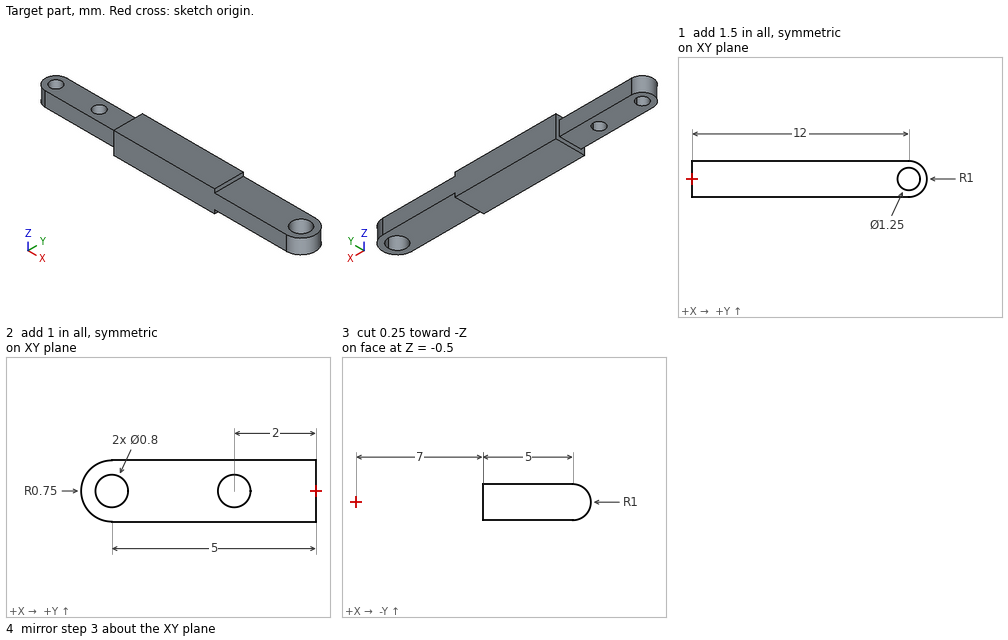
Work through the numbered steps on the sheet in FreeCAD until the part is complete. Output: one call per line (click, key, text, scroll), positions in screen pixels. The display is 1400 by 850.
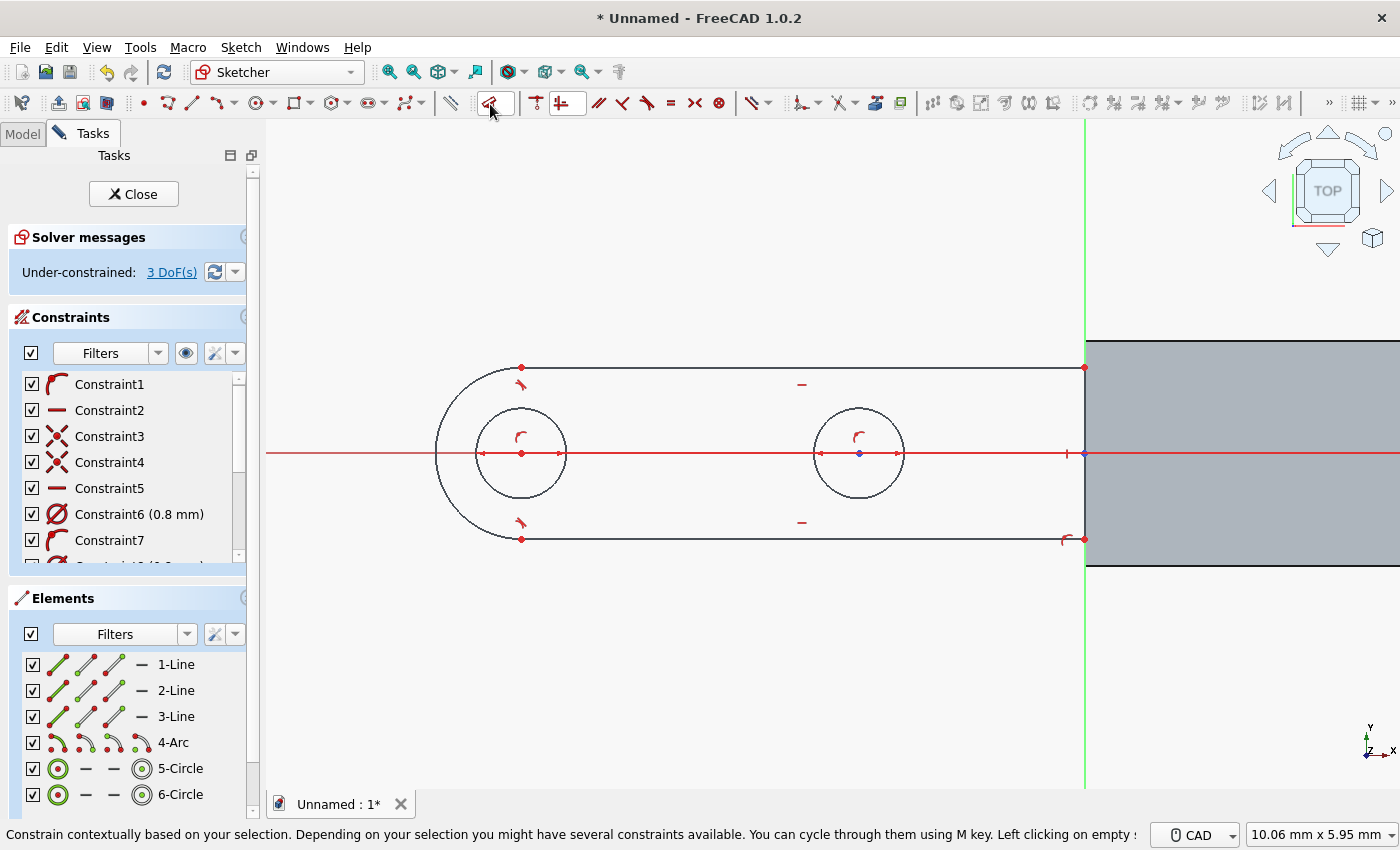
click(452, 403)
click(426, 384)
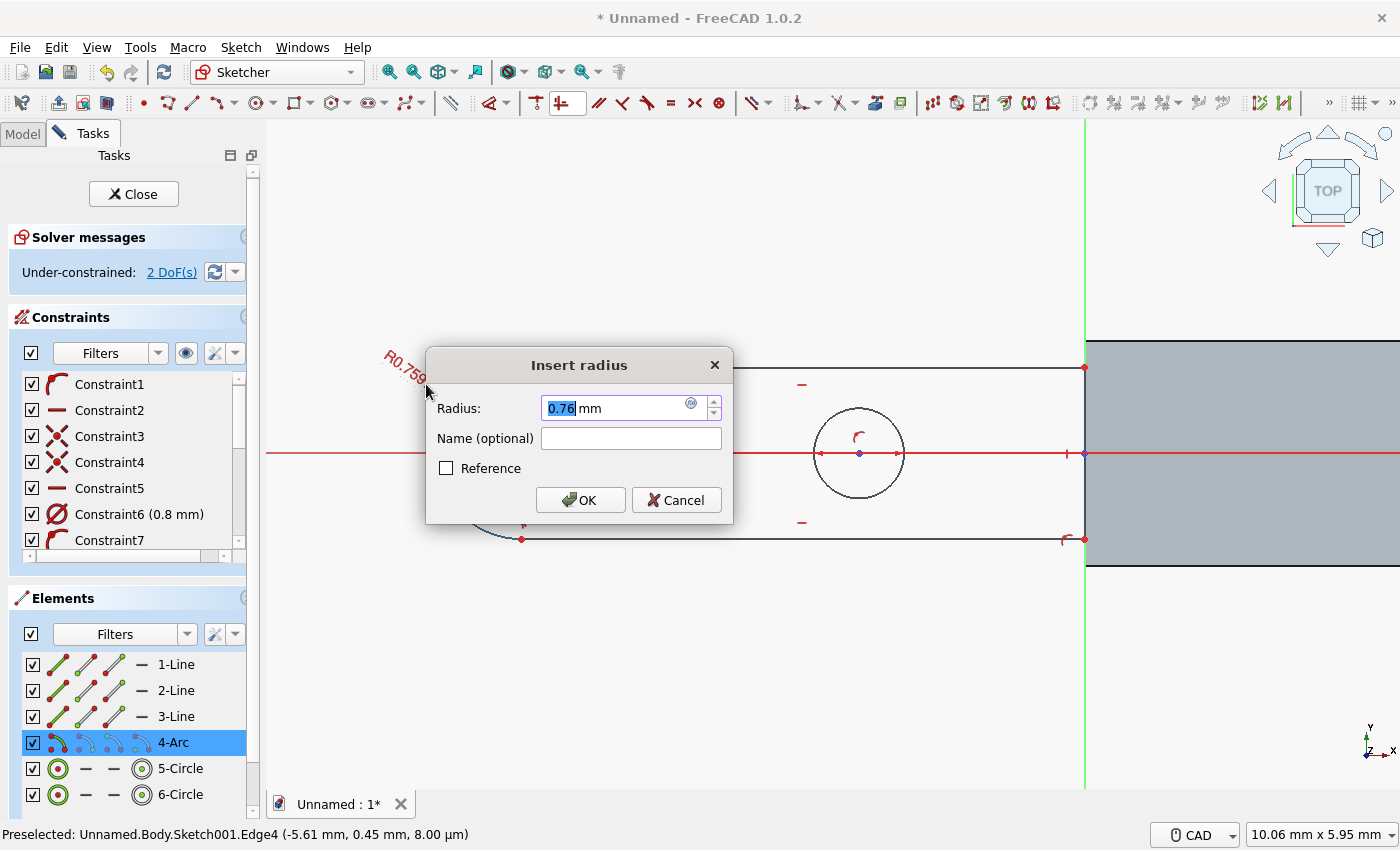
text(0.75)
key(Return)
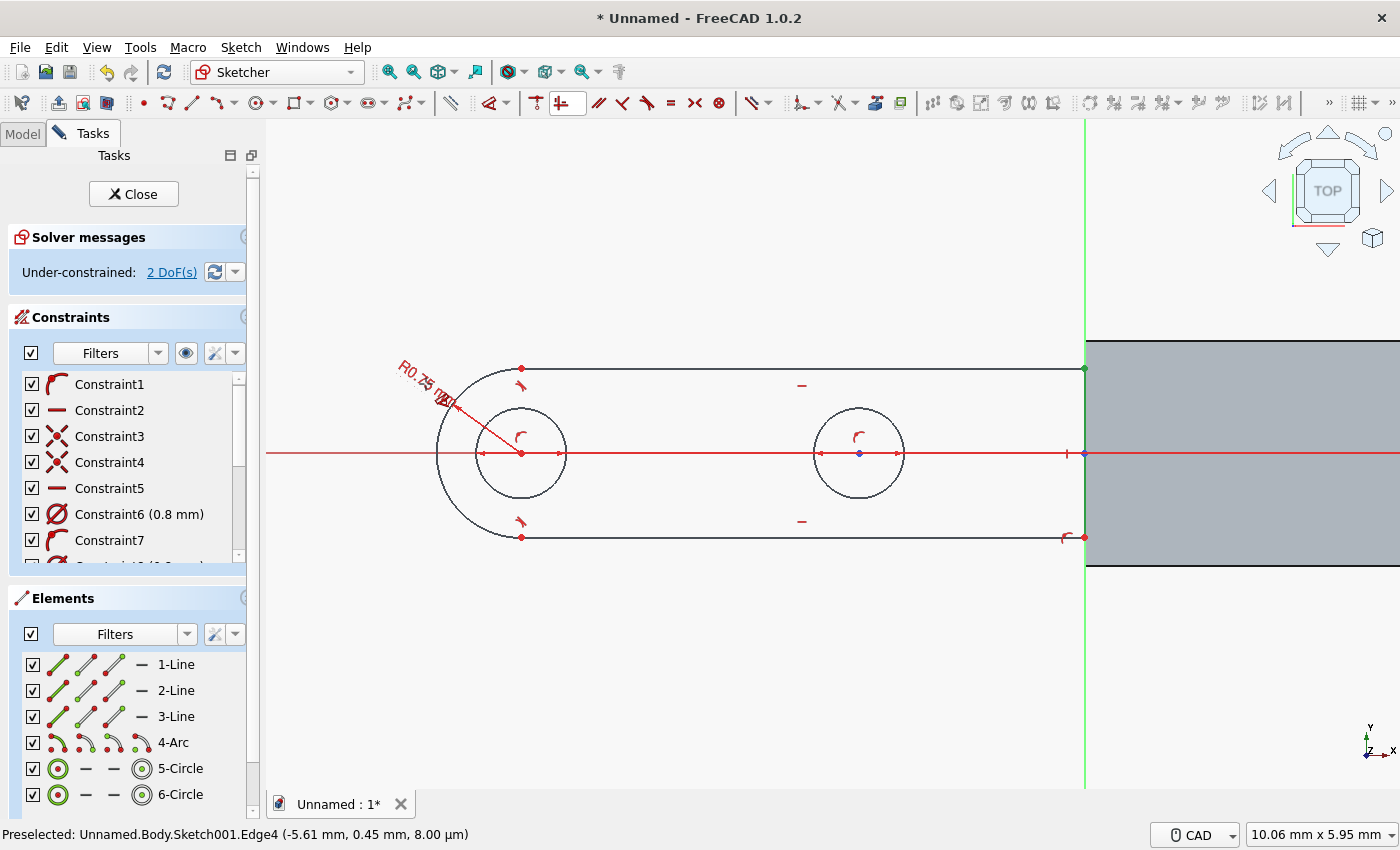
click(690, 538)
click(803, 572)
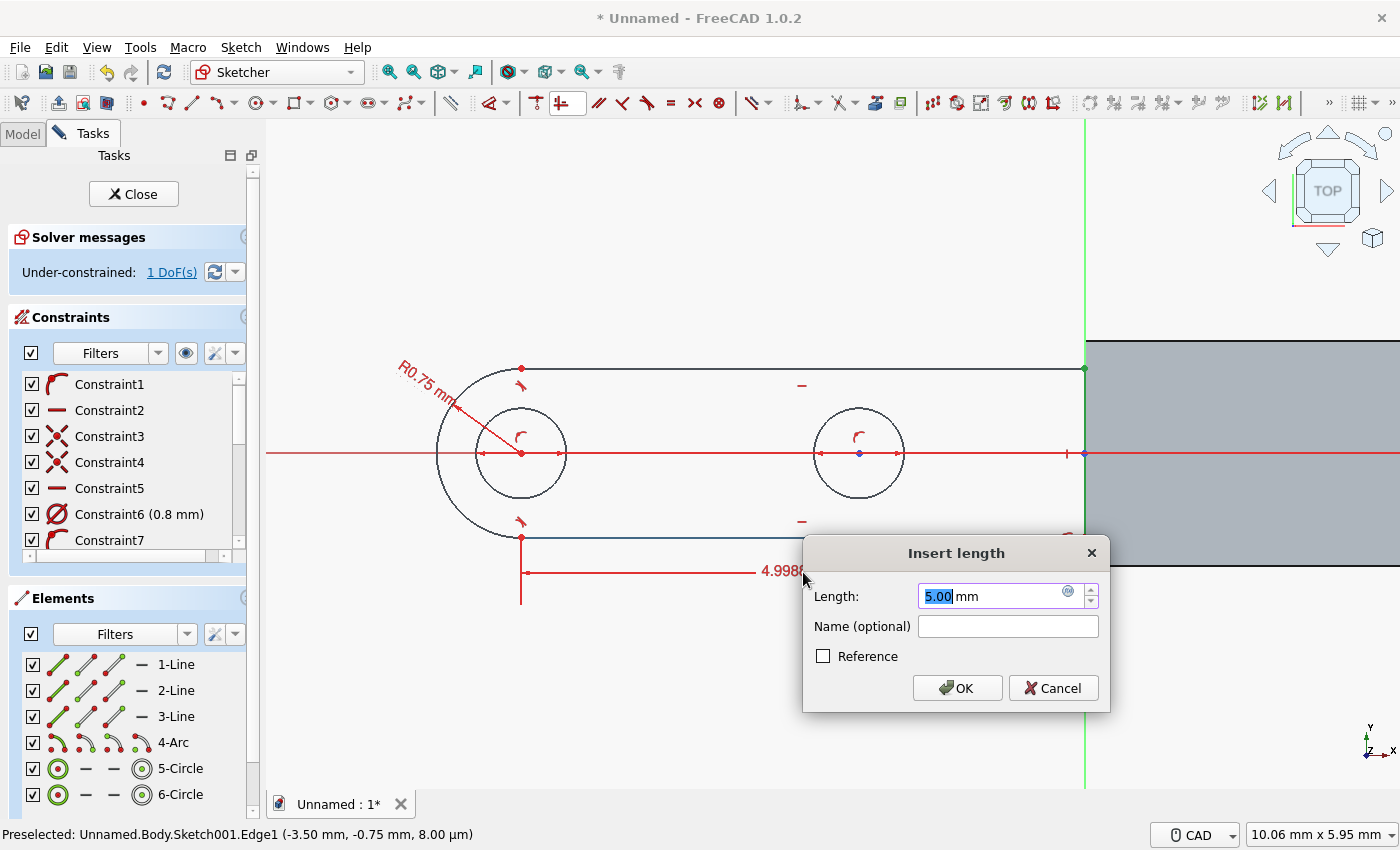
text(5)
key(Return)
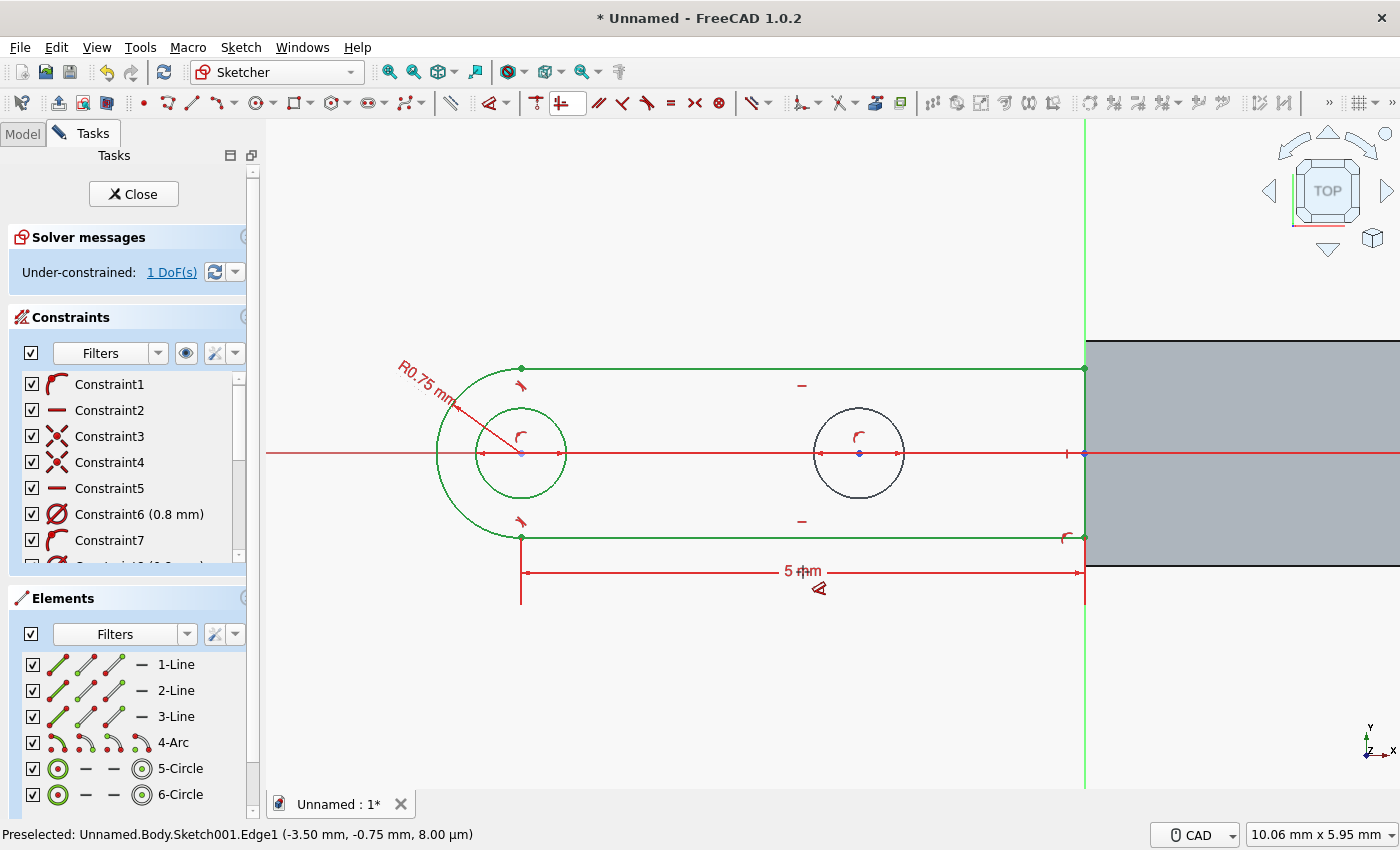
click(859, 453)
click(972, 487)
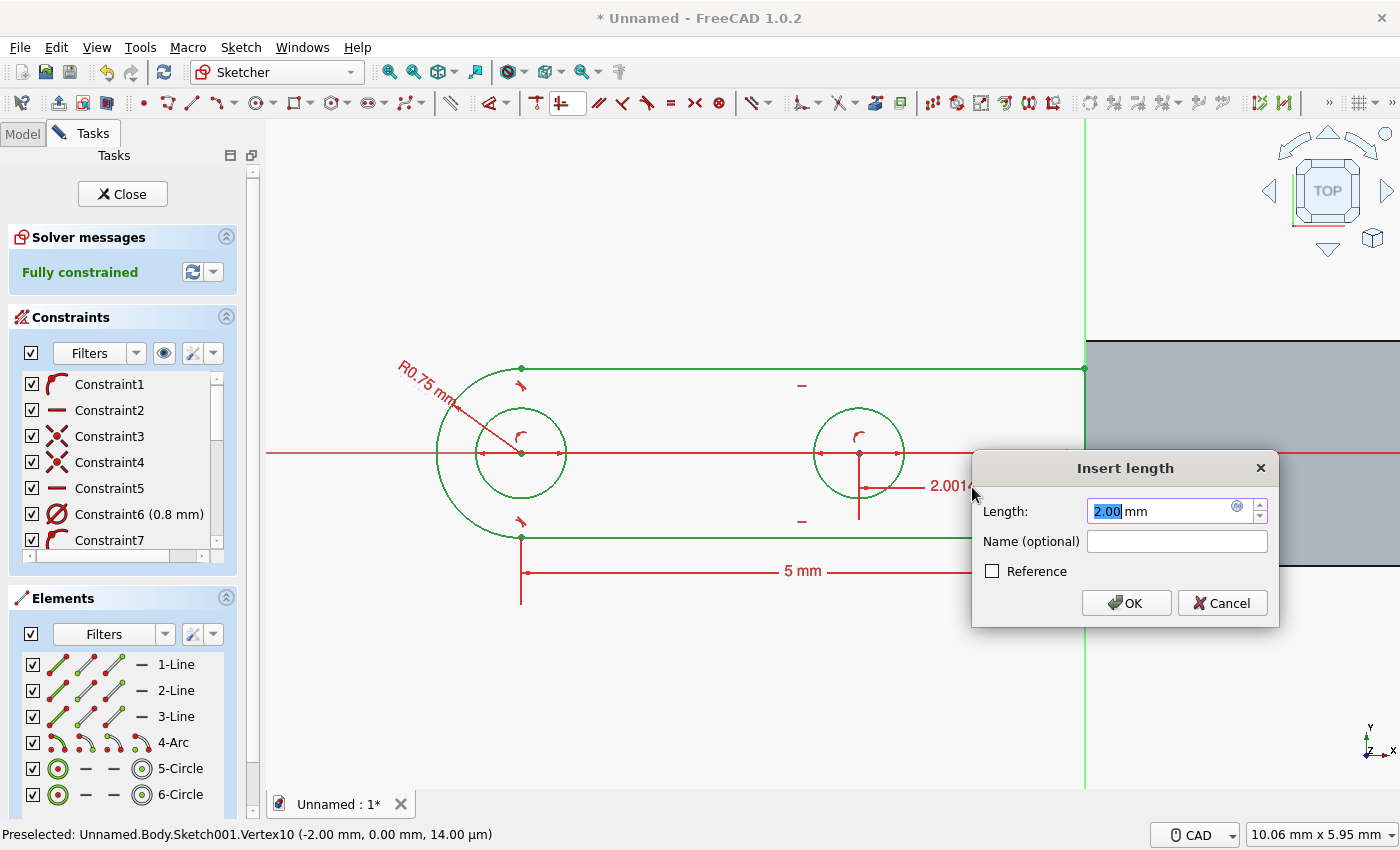
text(2)
key(Return)
key(Escape)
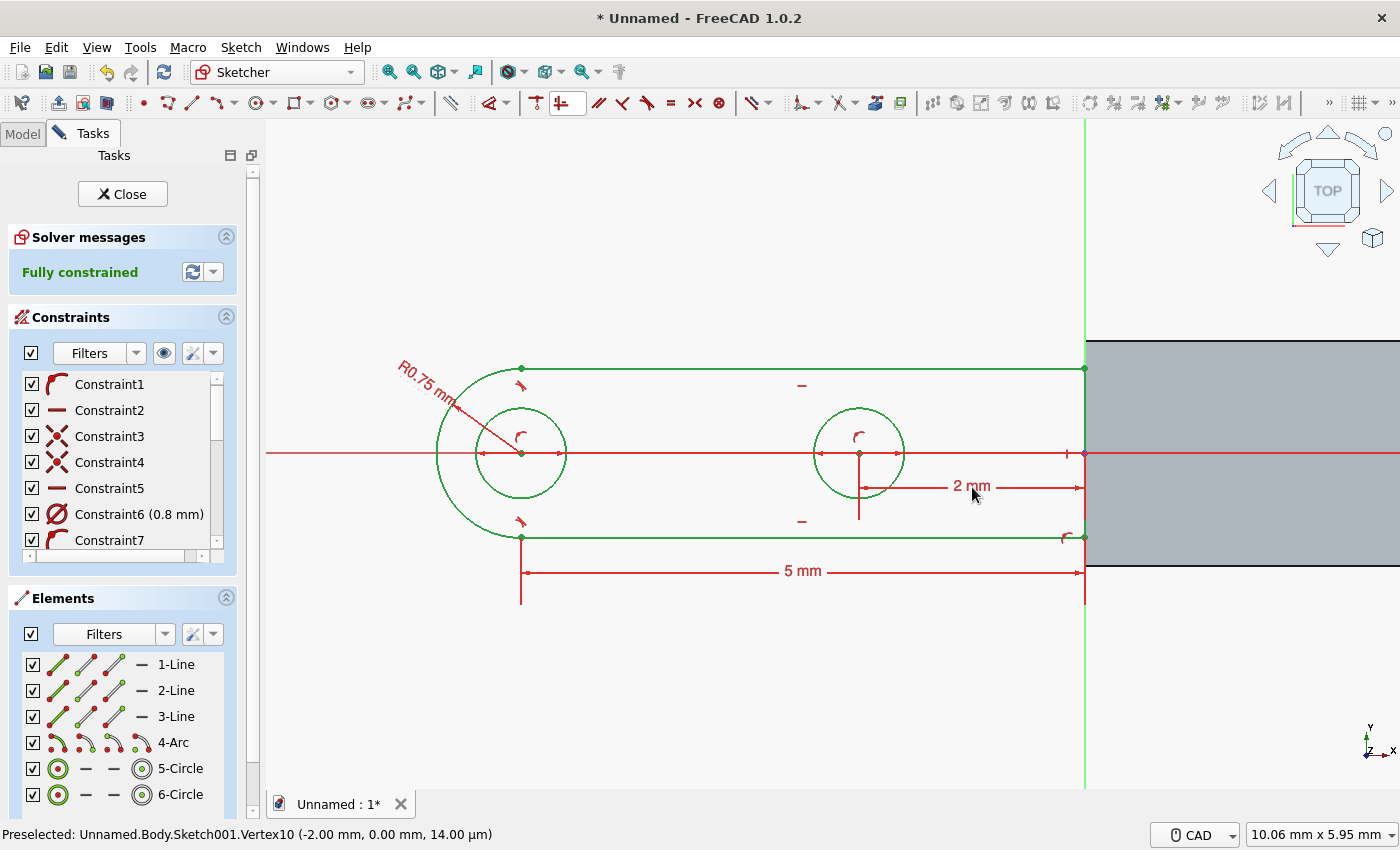
click(123, 194)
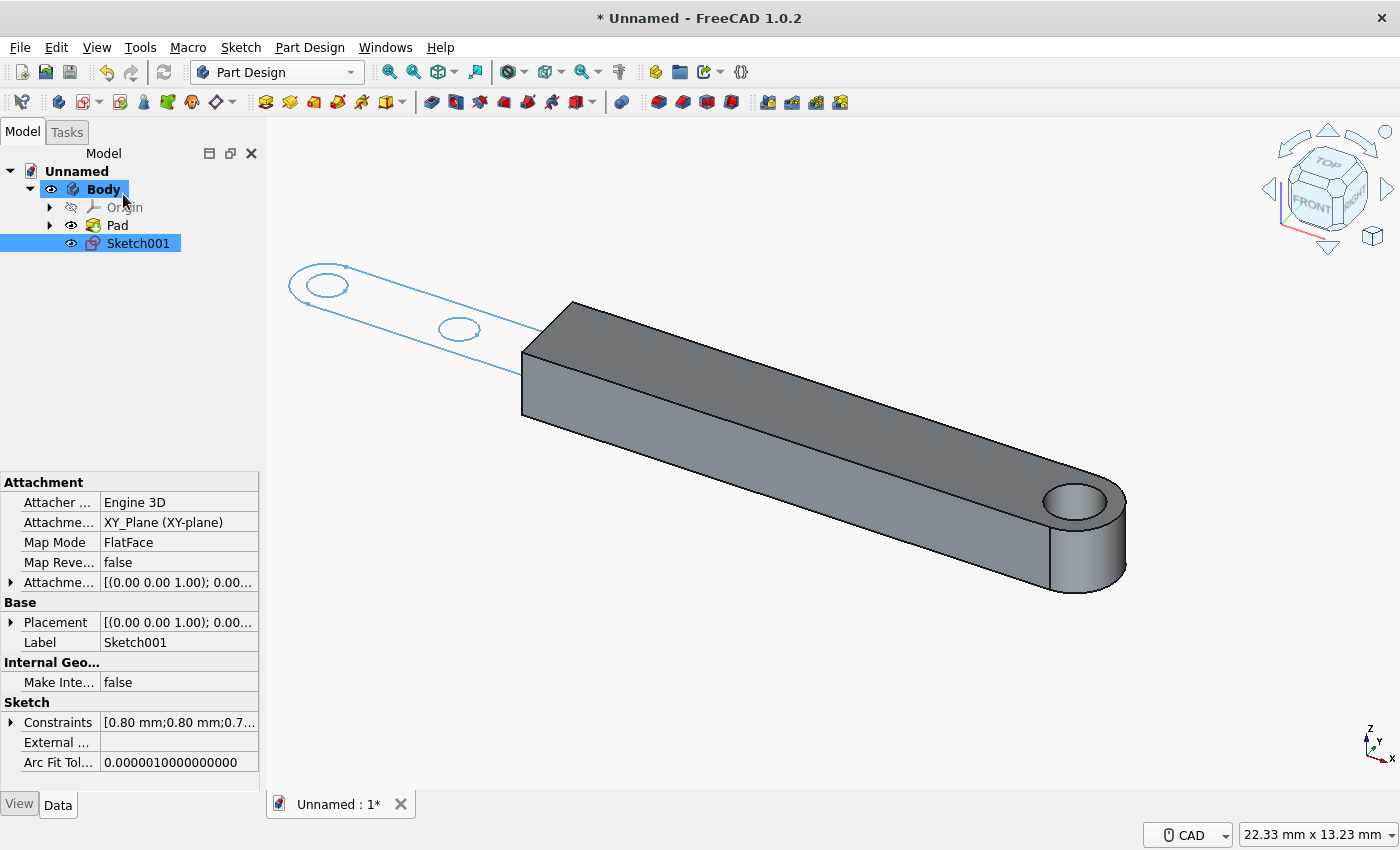
click(266, 102)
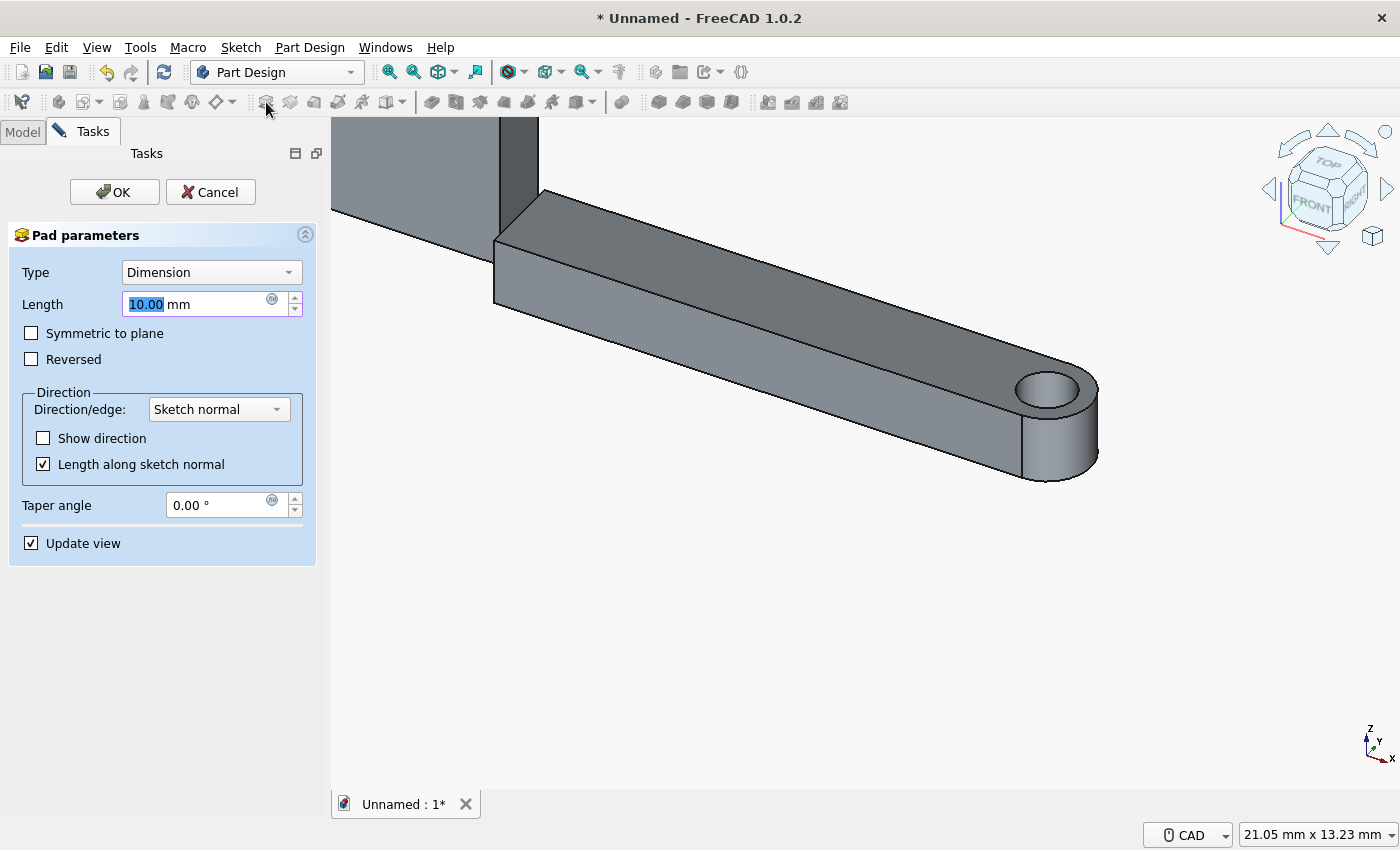
text(1)
key(Tab)